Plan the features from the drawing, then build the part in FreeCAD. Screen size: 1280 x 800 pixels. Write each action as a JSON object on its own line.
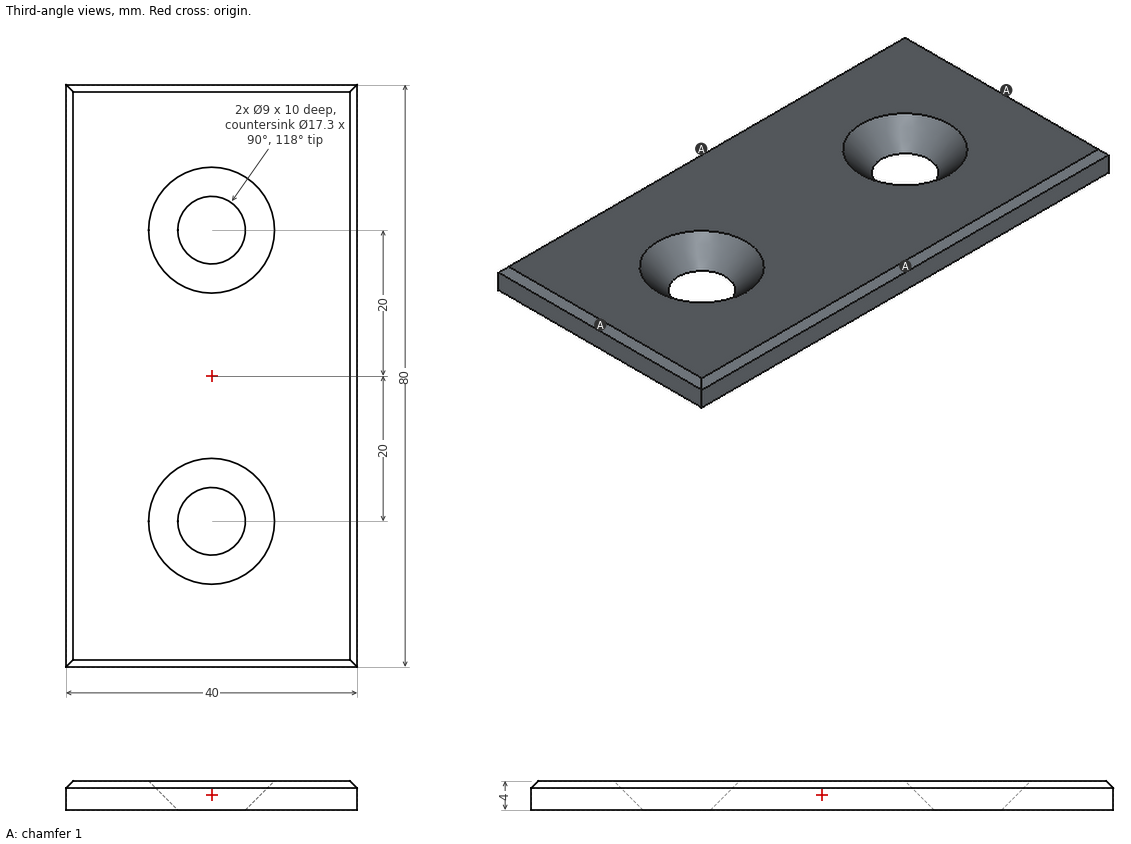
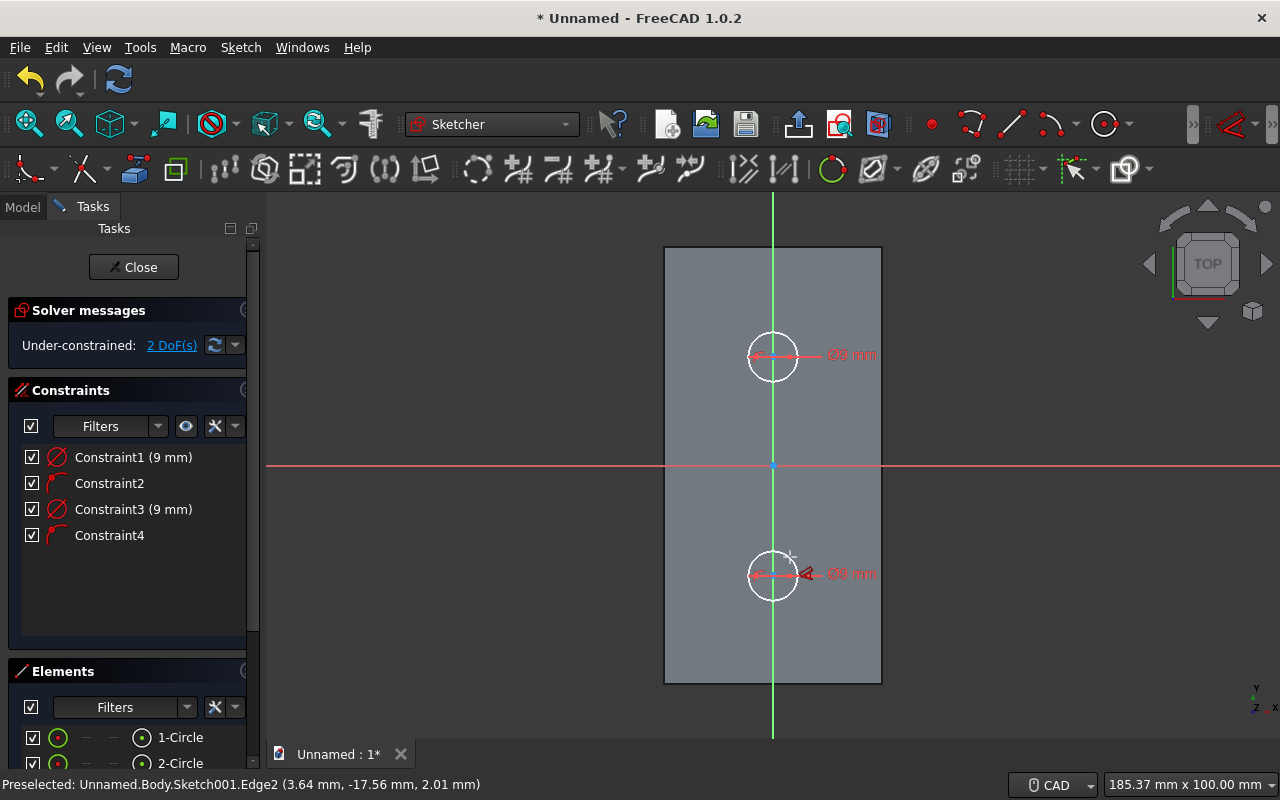
{"action": "left_click", "coordinate": [773, 357]}
{"action": "left_click", "coordinate": [807, 411]}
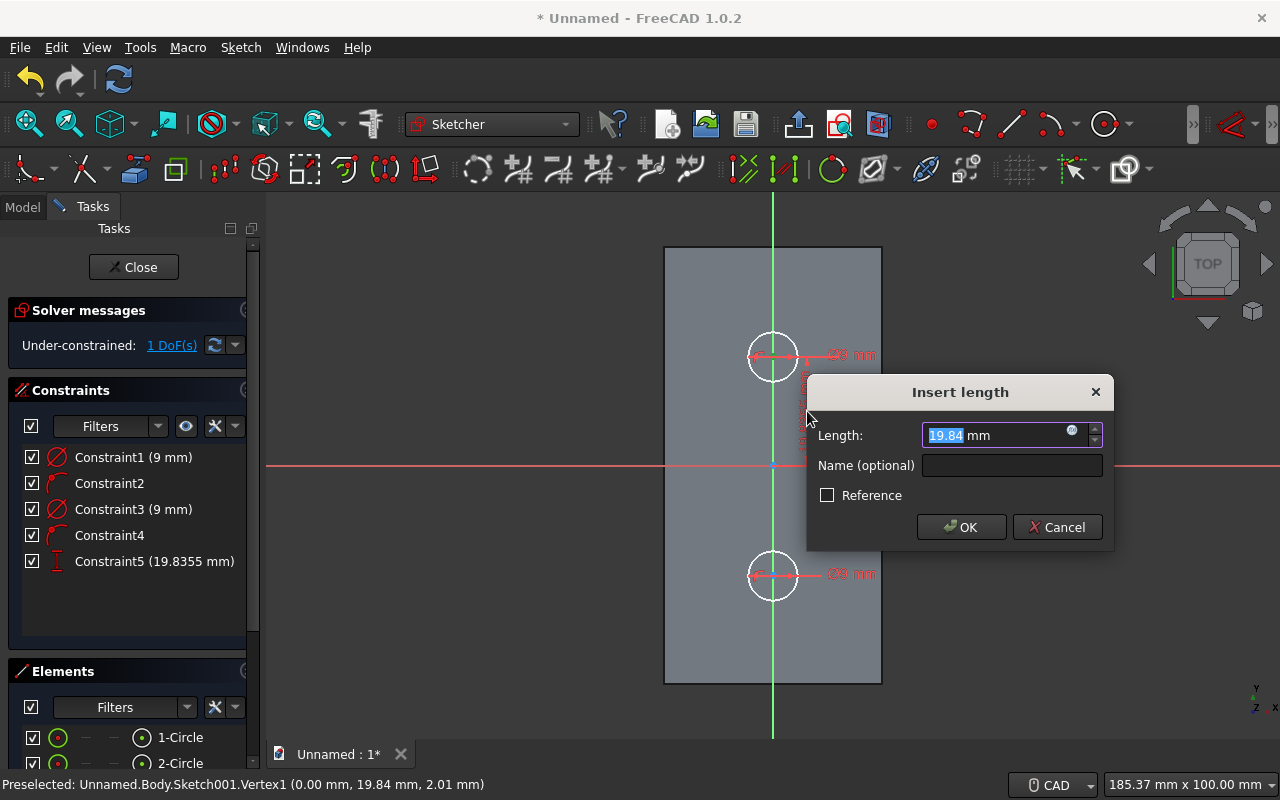
{"action": "type", "text": "20"}
{"action": "key", "text": "Return"}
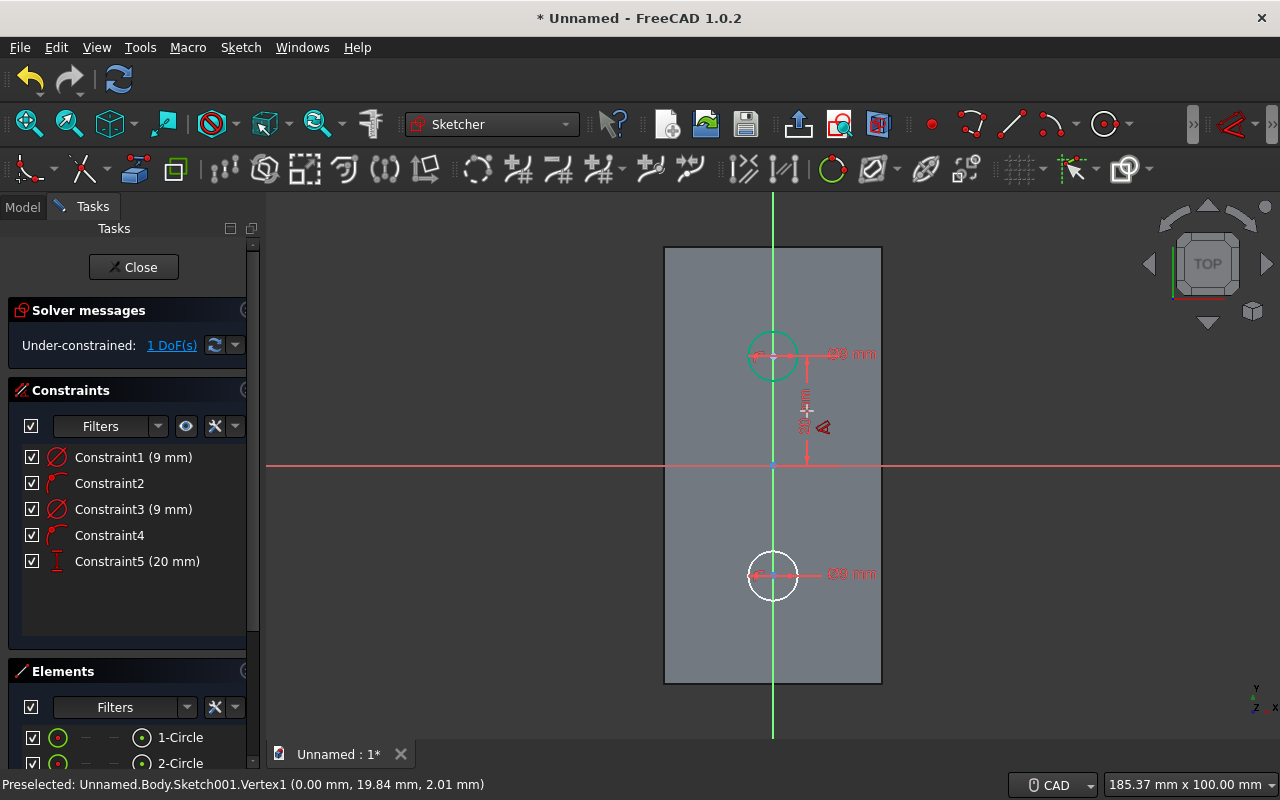
{"action": "left_click", "coordinate": [773, 576]}
{"action": "left_click", "coordinate": [807, 521]}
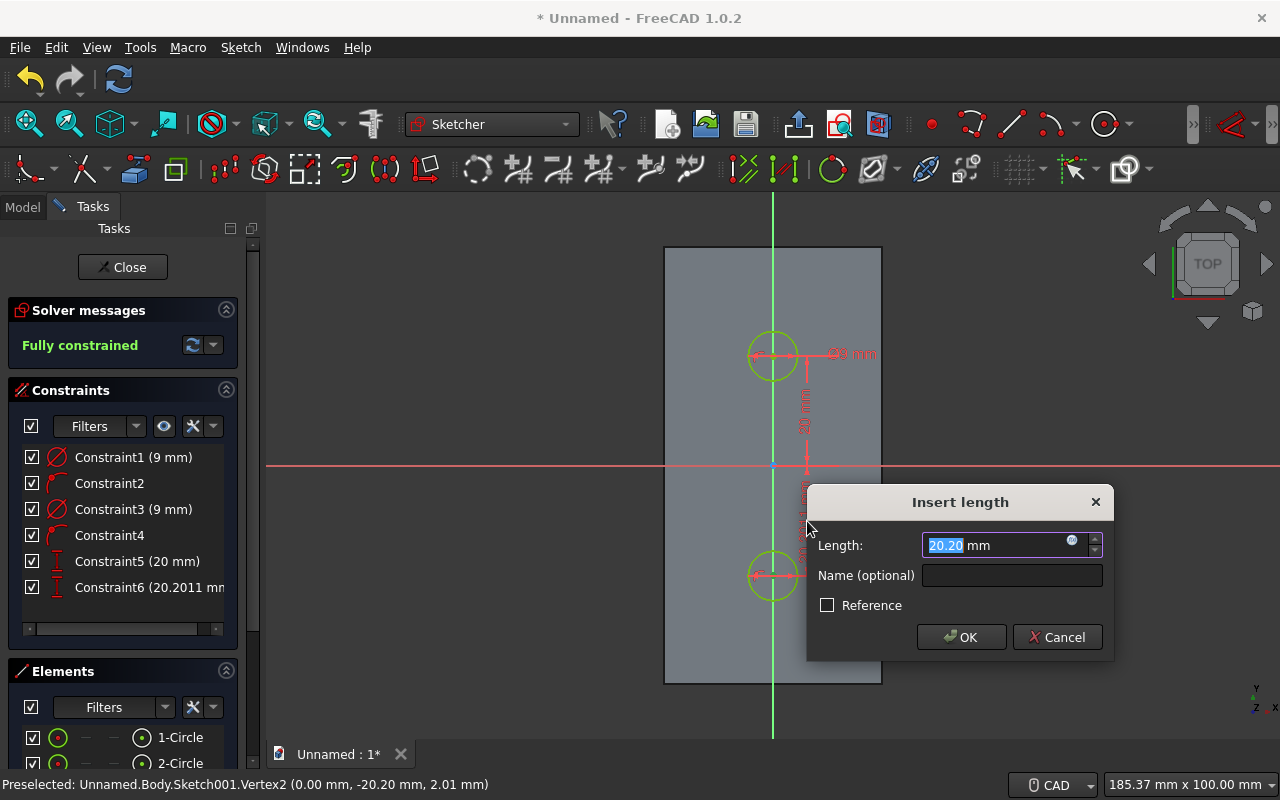
{"action": "type", "text": "20"}
{"action": "key", "text": "Return"}
{"action": "key", "text": "Escape"}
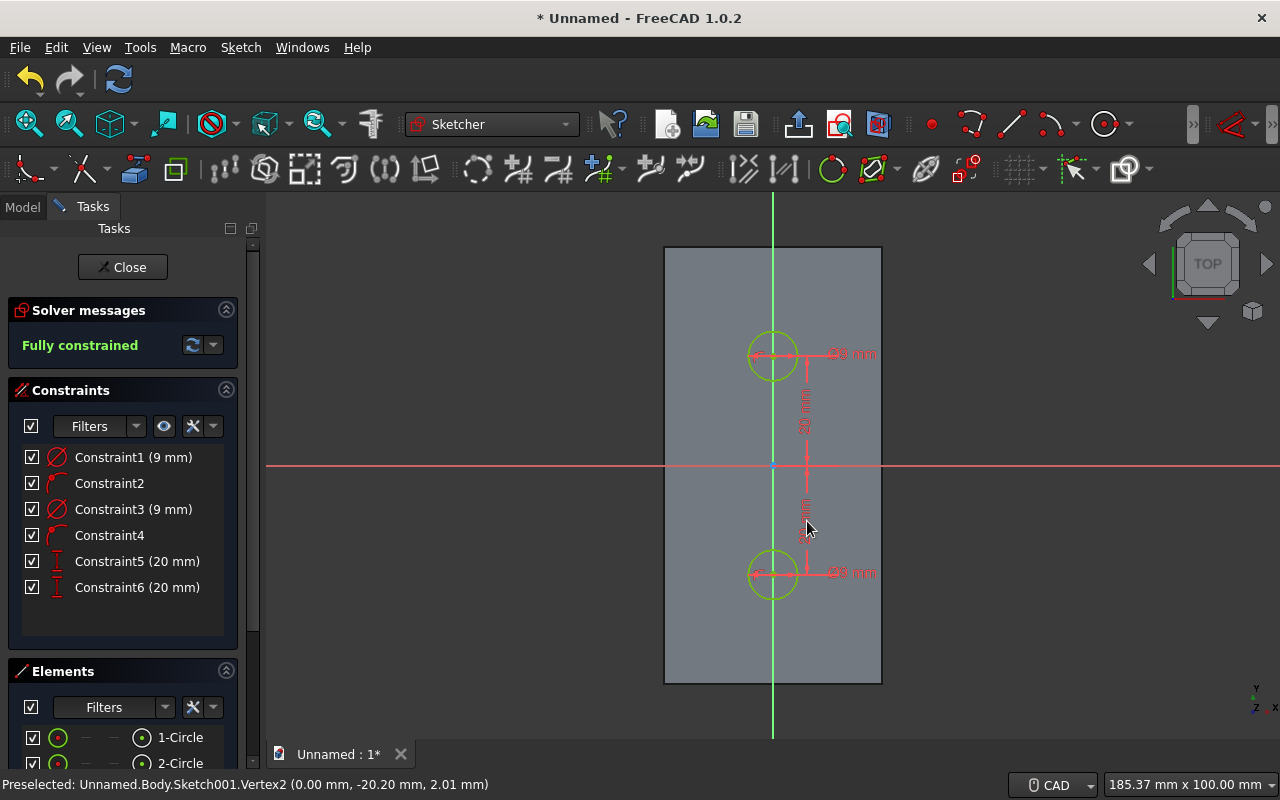
{"action": "left_click", "coordinate": [123, 267]}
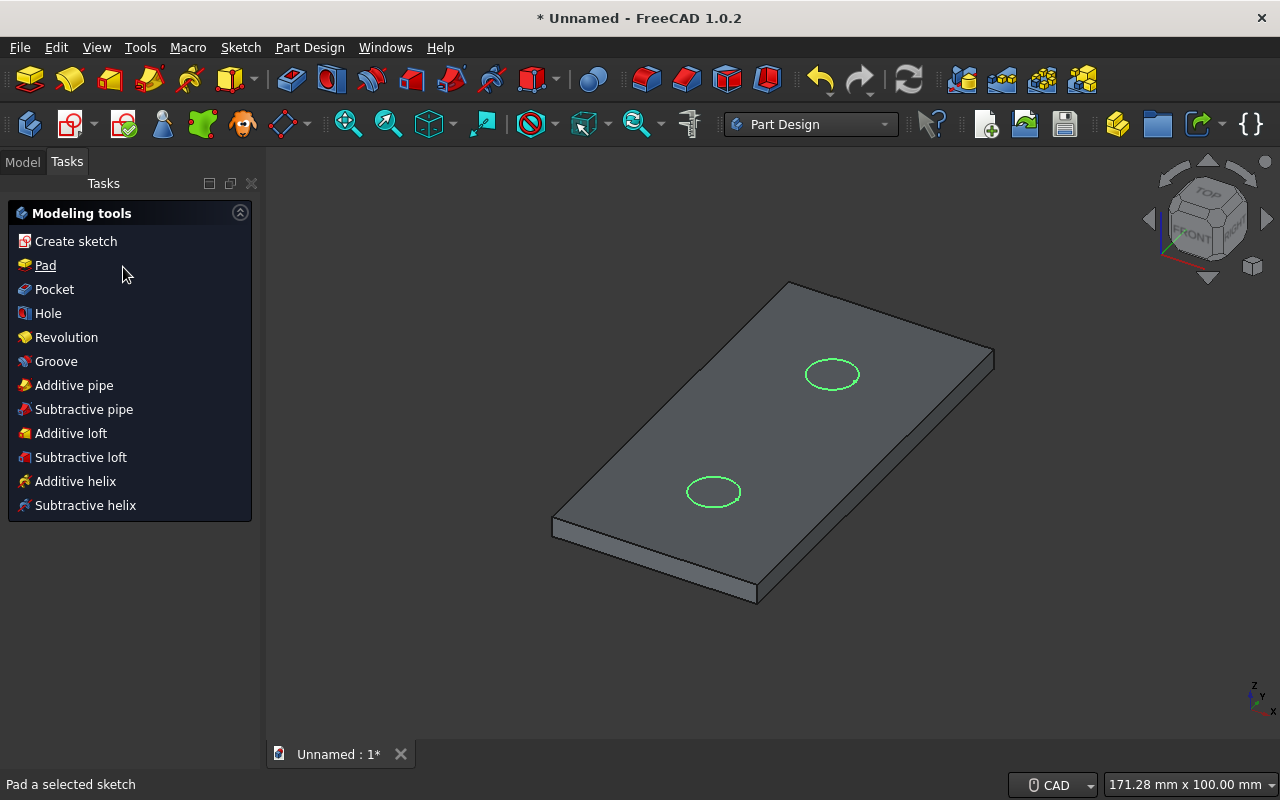
{"action": "left_click", "coordinate": [332, 80]}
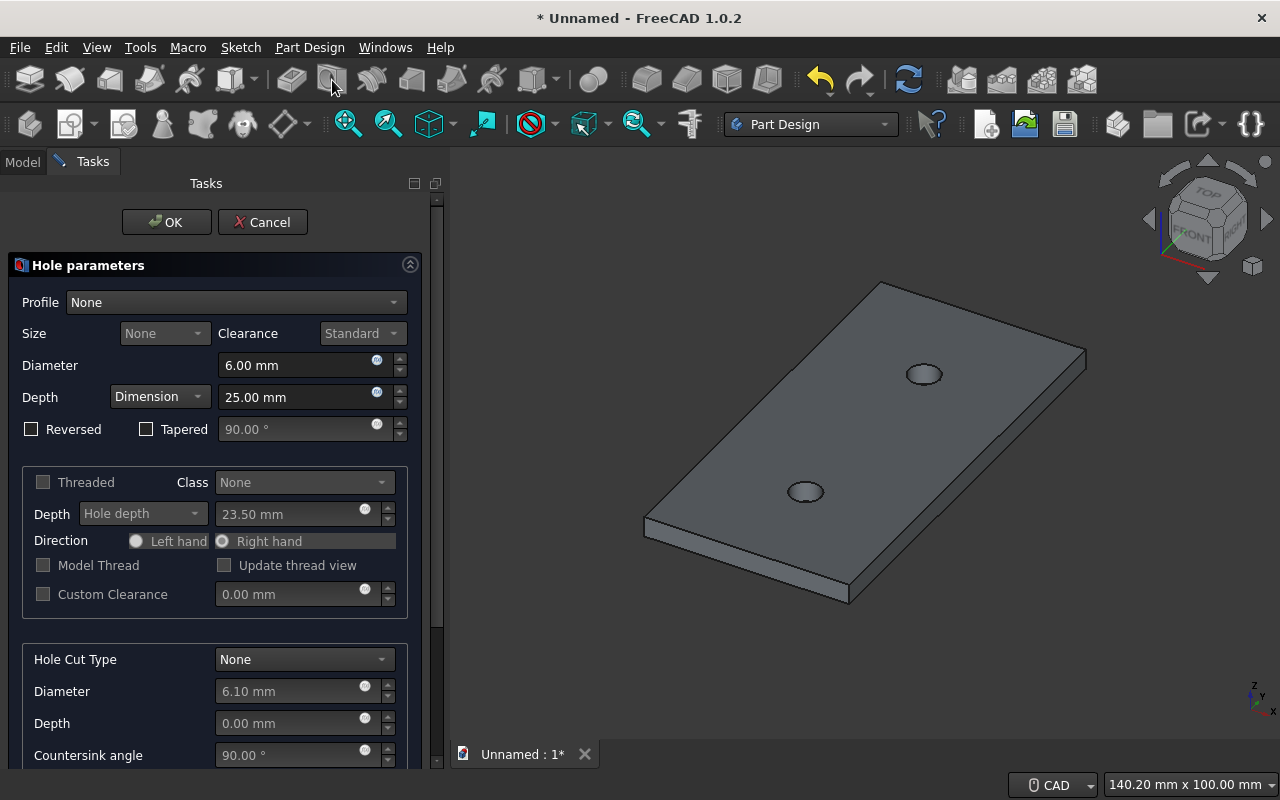
{"action": "triple_click", "coordinate": [305, 365]}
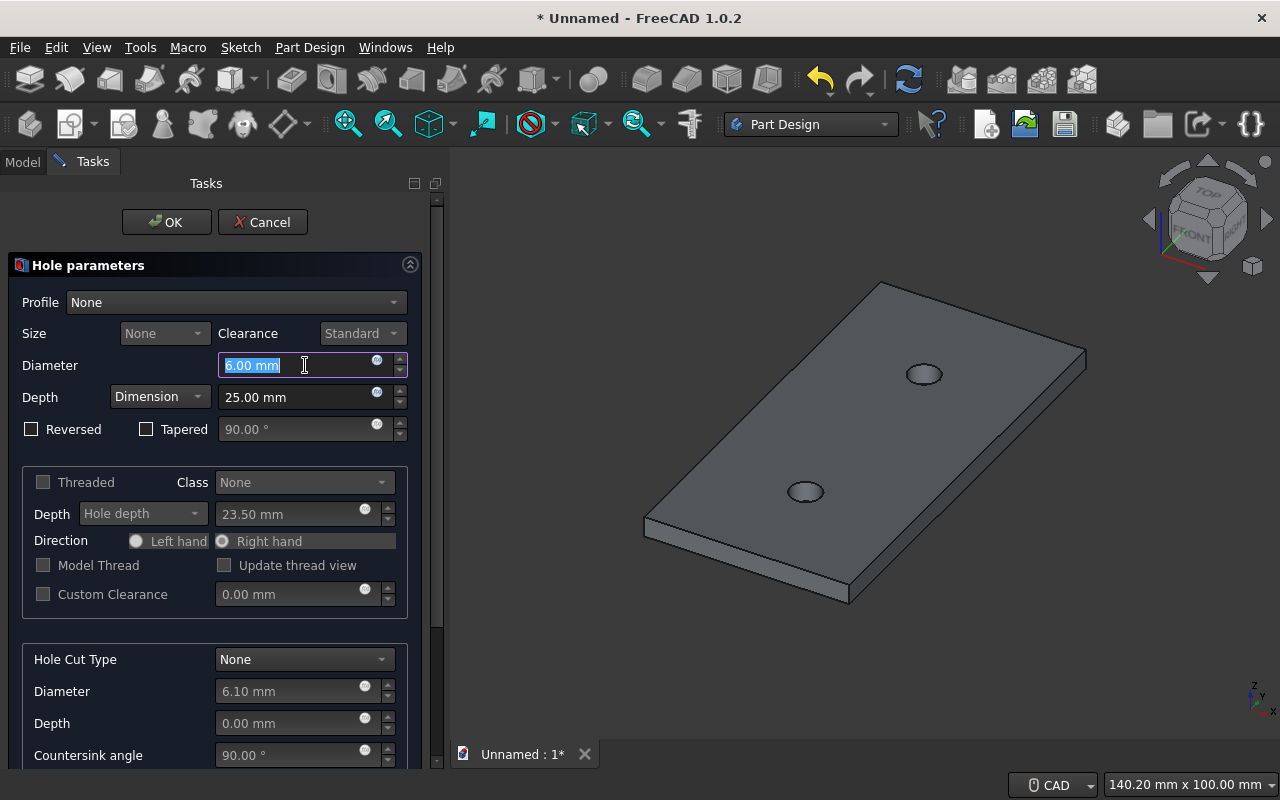
{"action": "type", "text": "9"}
{"action": "key", "text": "Tab"}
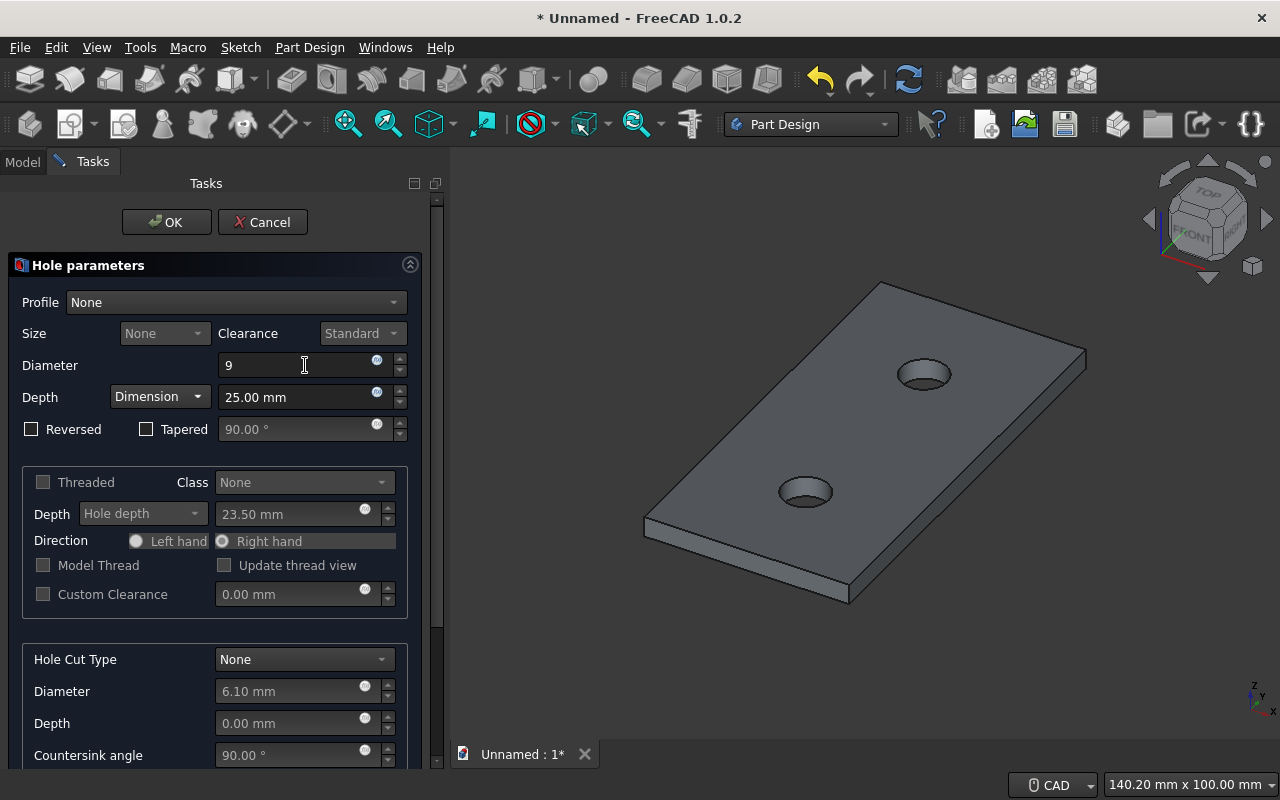
{"action": "triple_click", "coordinate": [305, 397]}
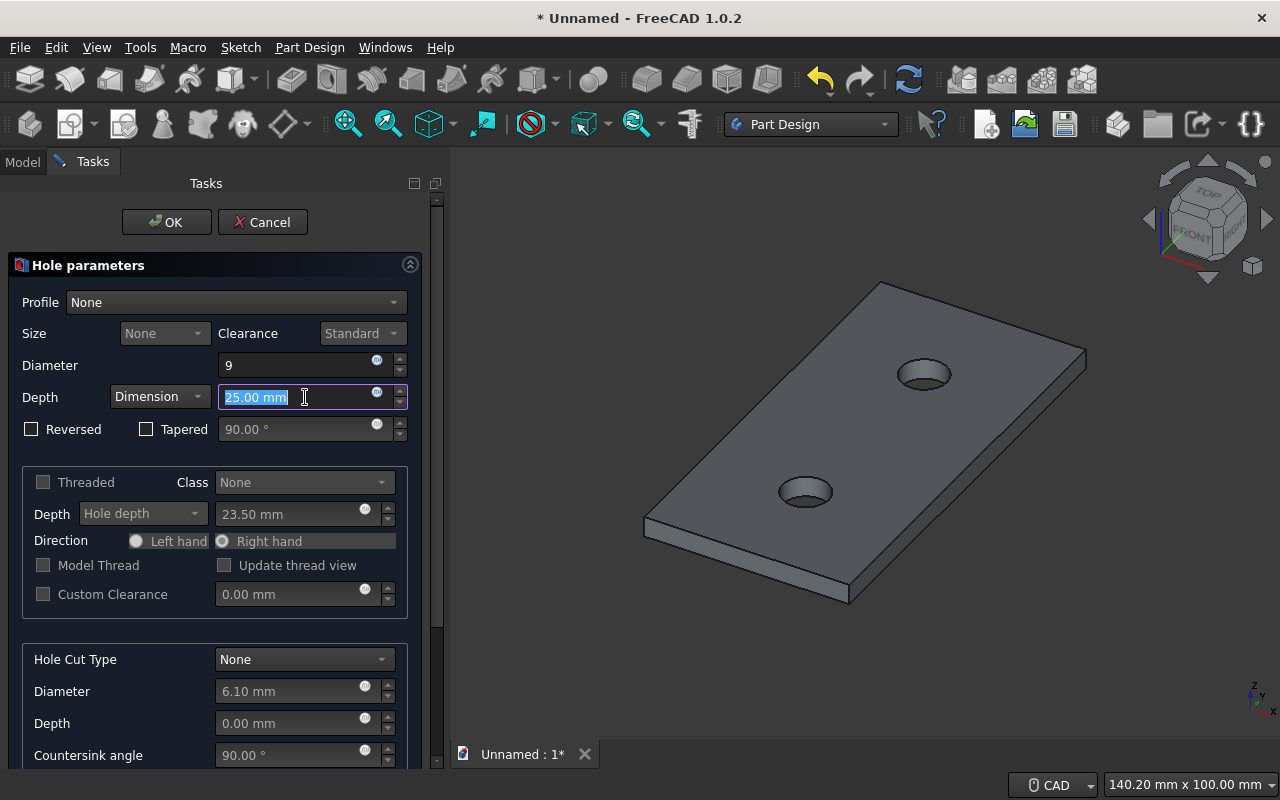
{"action": "type", "text": "10"}
{"action": "key", "text": "Tab"}